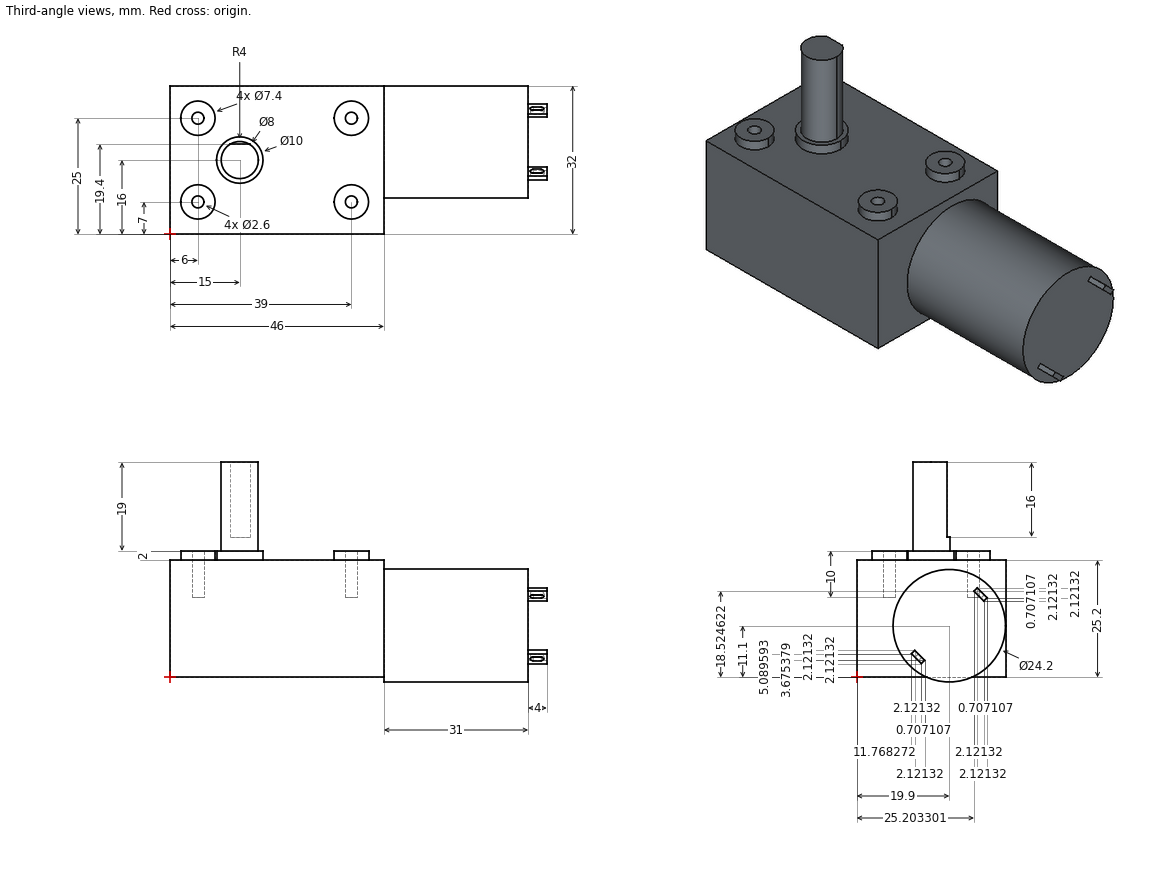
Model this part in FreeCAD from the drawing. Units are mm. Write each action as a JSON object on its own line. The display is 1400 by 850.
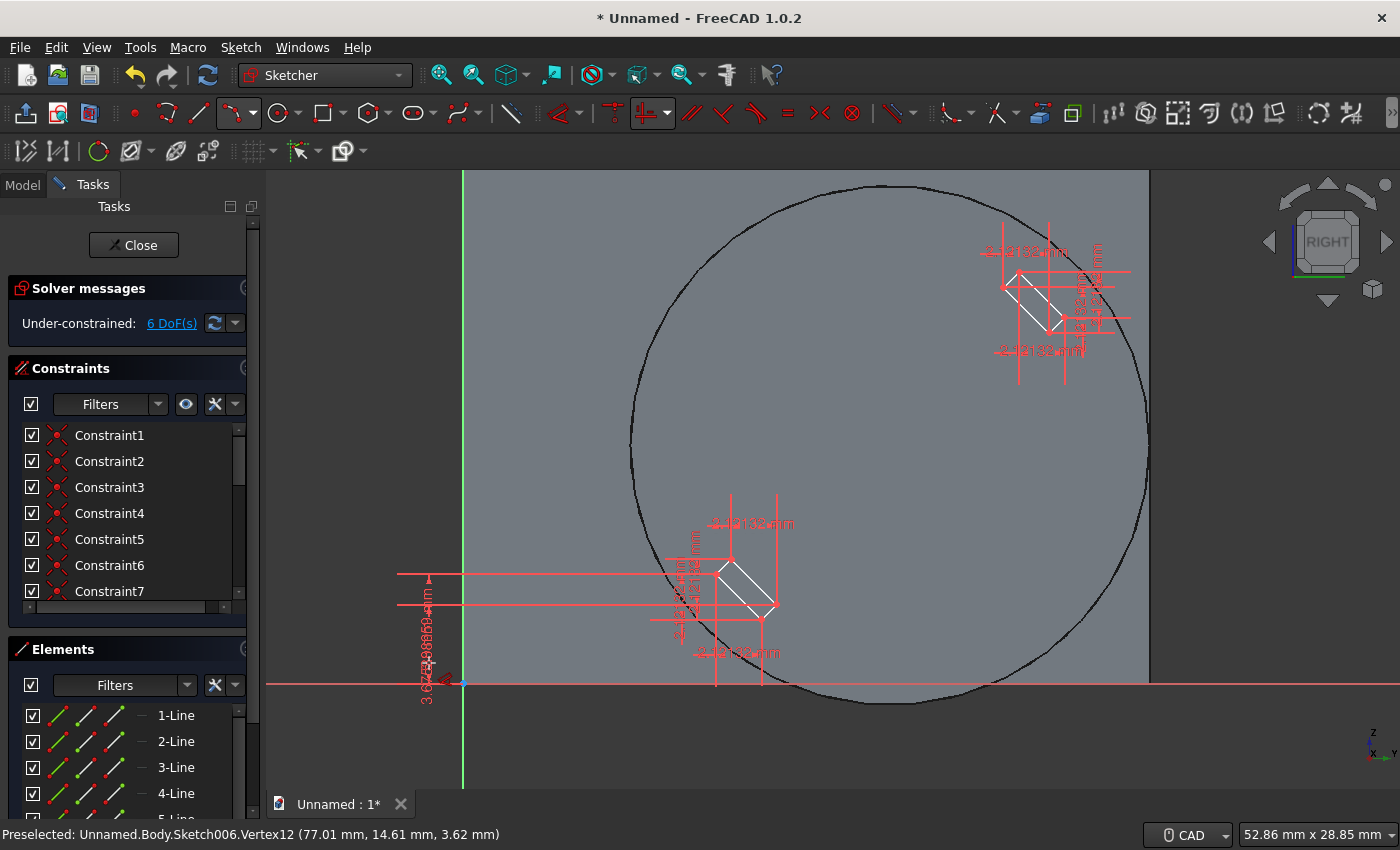
{"action": "scroll", "coordinate": [1057, 326], "scroll_direction": "up", "scroll_amount": 5}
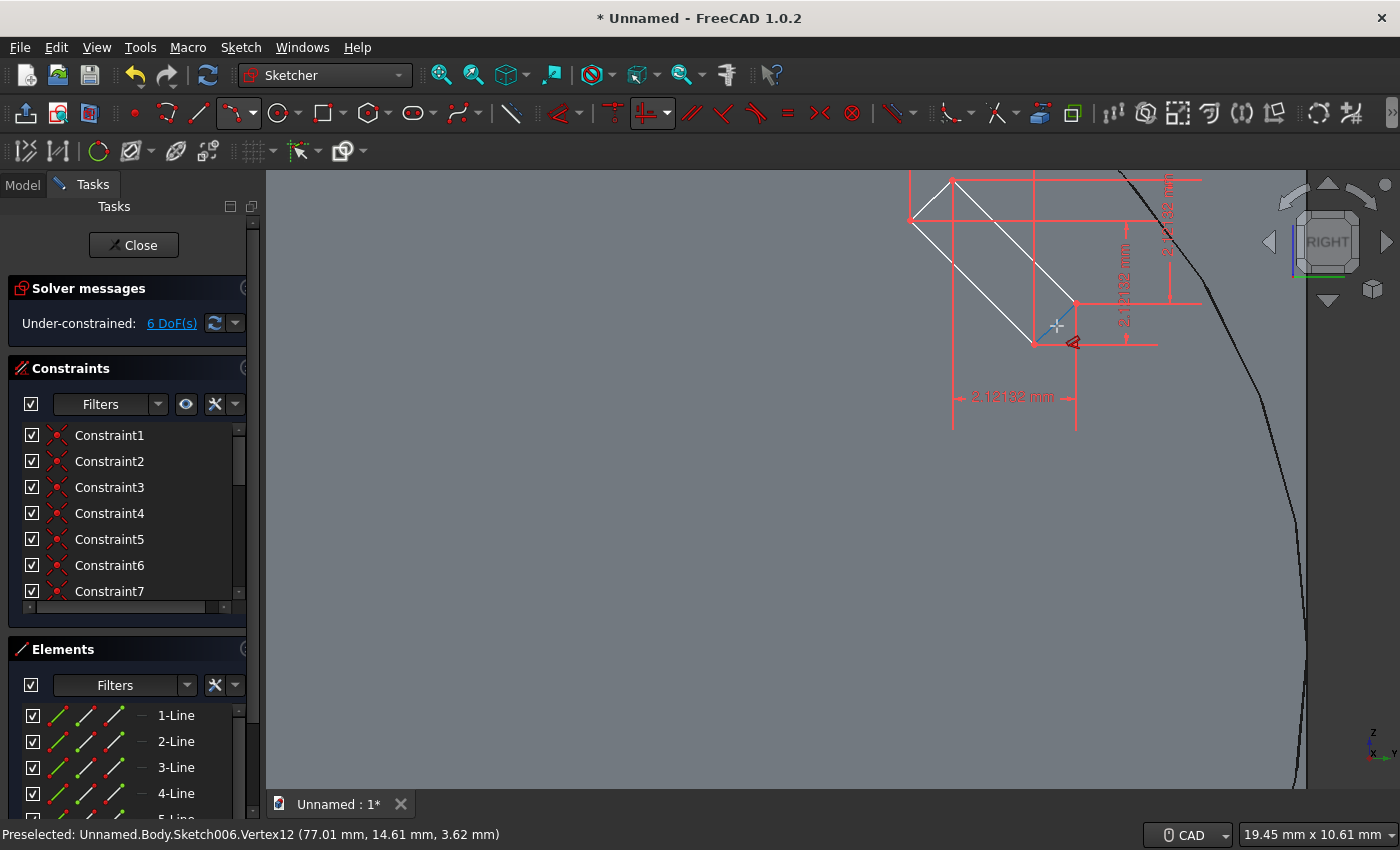
{"action": "left_click", "coordinate": [1055, 324]}
{"action": "left_click", "coordinate": [1055, 246]}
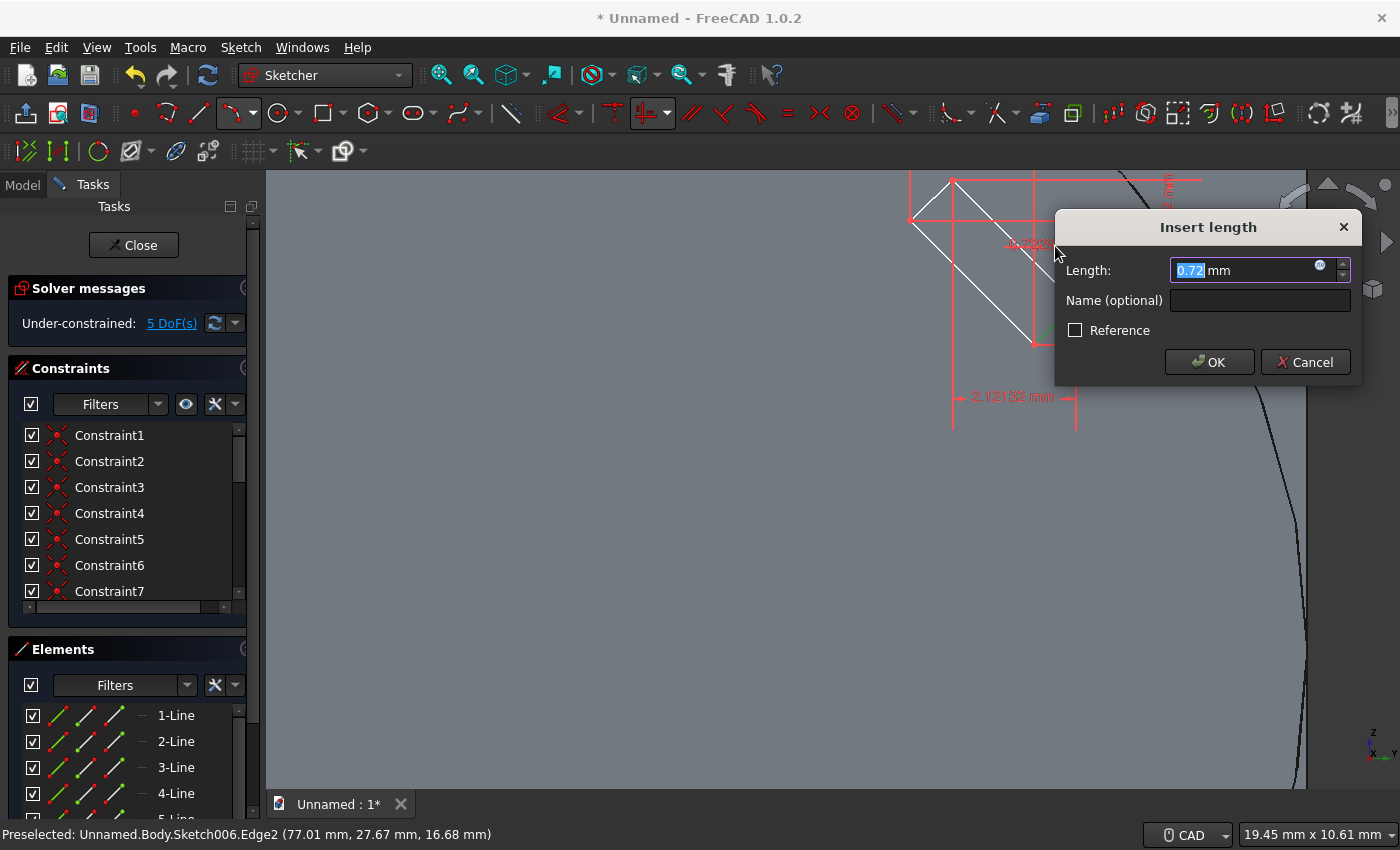
{"action": "type", "text": "0.707107"}
{"action": "key", "text": "Return"}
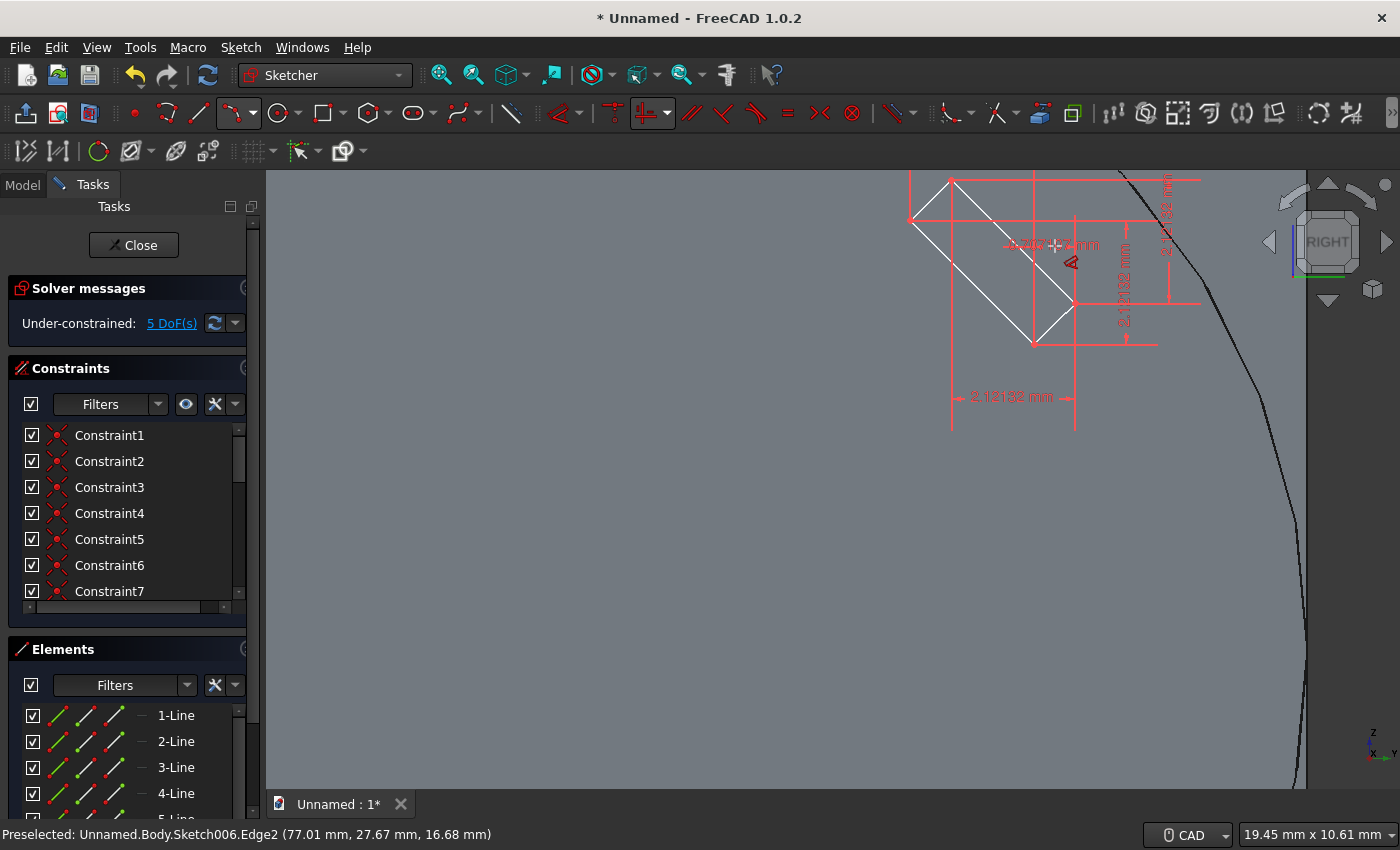
{"action": "left_click", "coordinate": [1046, 332]}
{"action": "left_click", "coordinate": [1109, 324]}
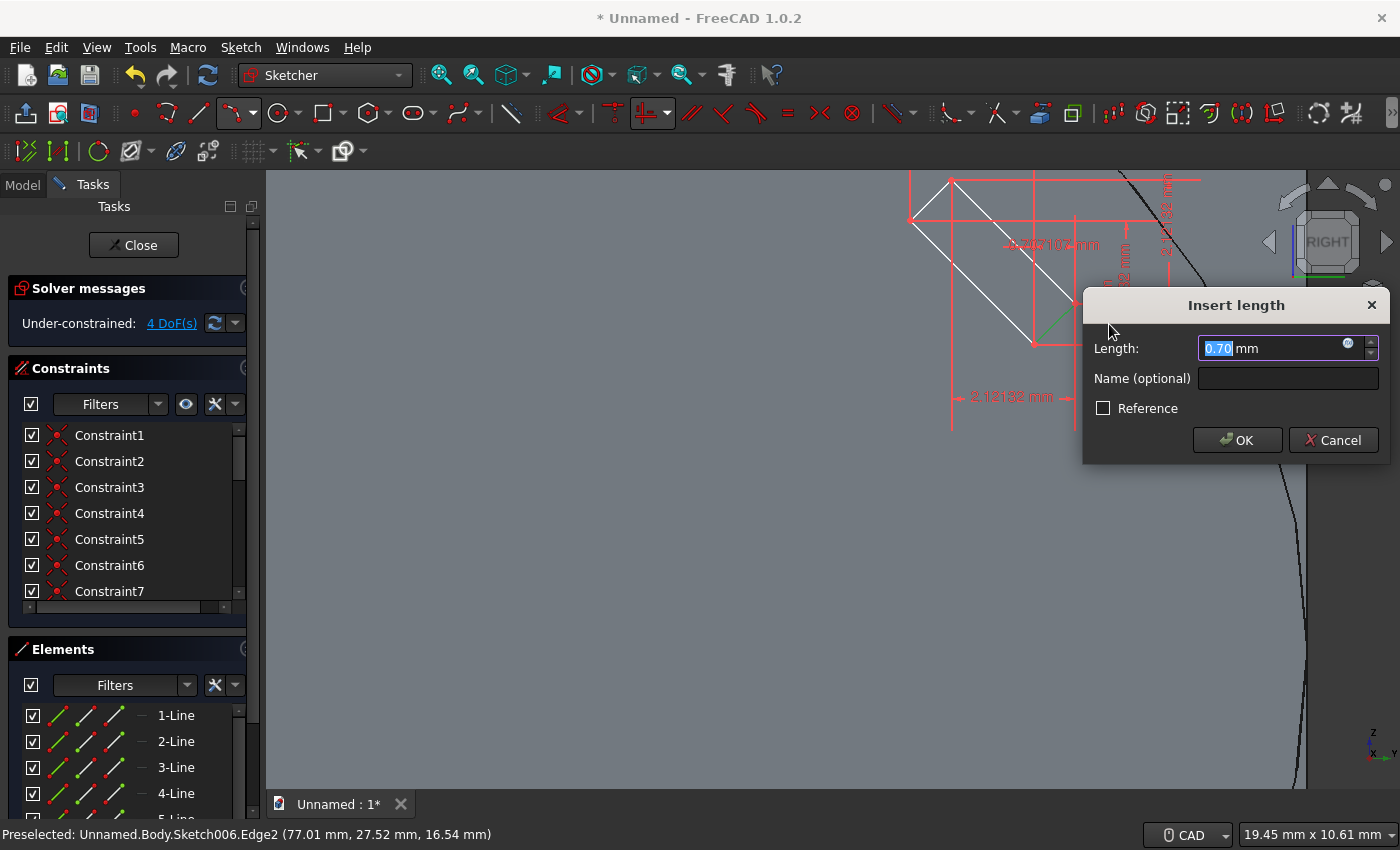
{"action": "type", "text": "0.707107"}
{"action": "key", "text": "Return"}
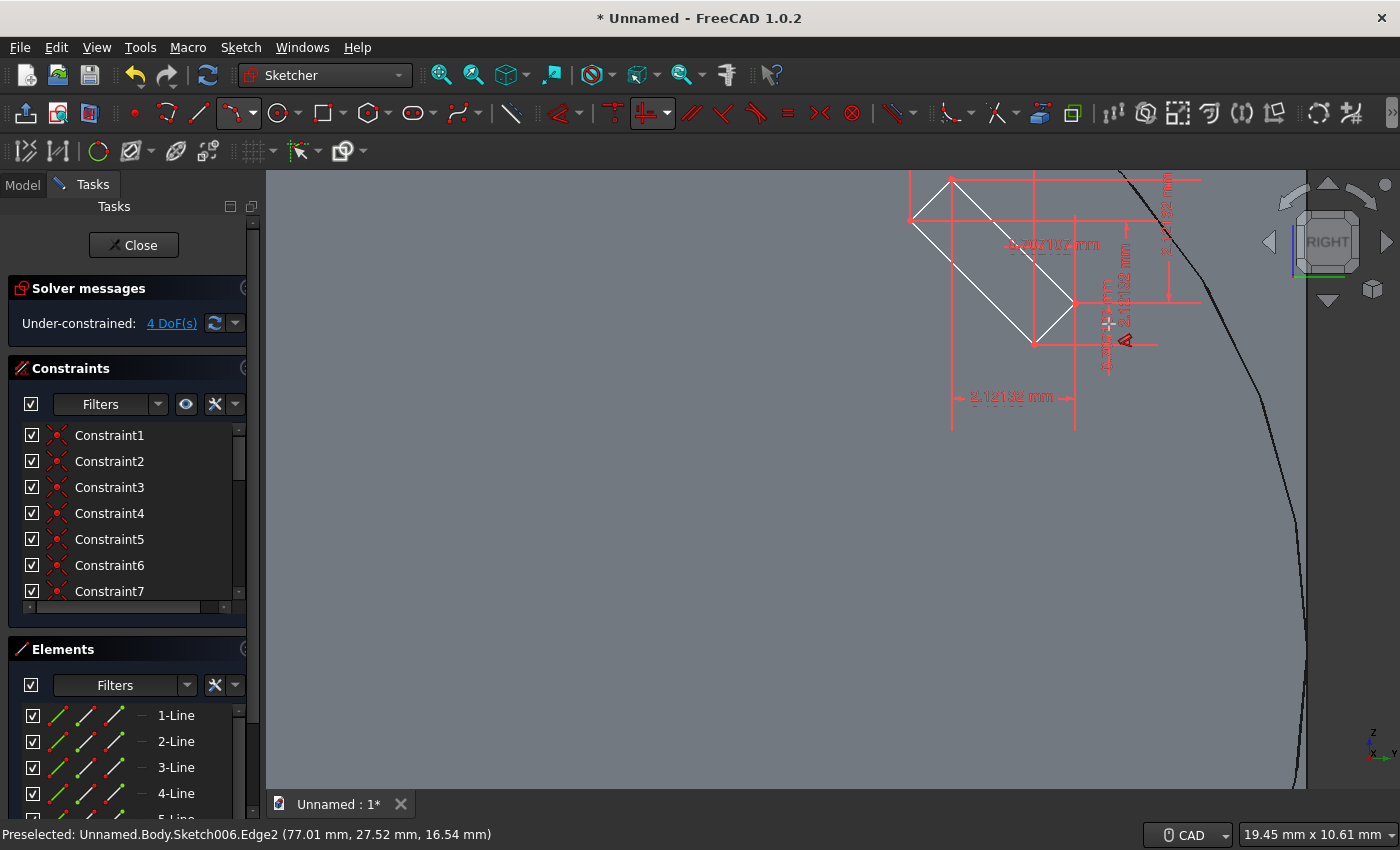
{"action": "scroll", "coordinate": [1059, 330], "scroll_direction": "down", "scroll_amount": 5}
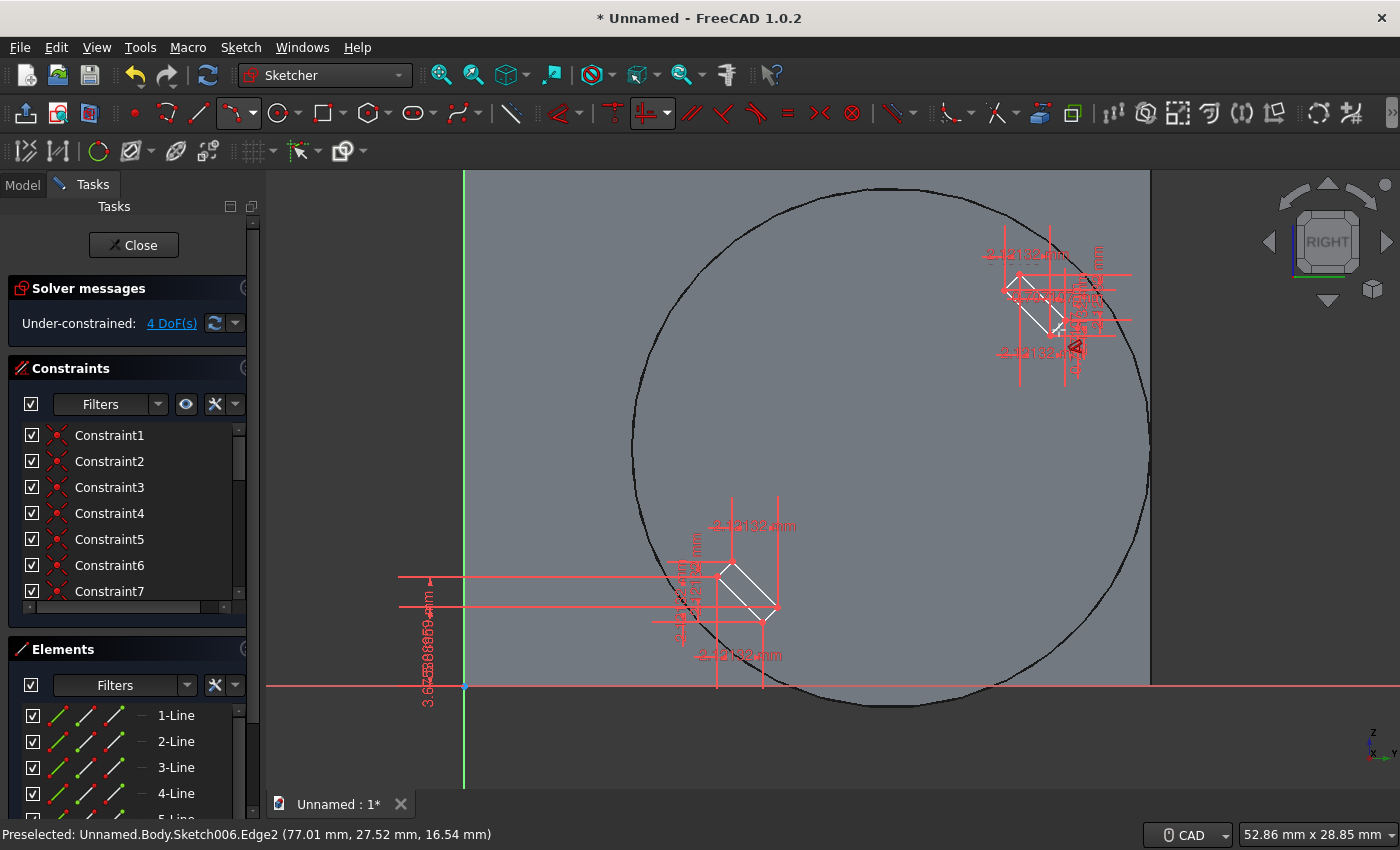
{"action": "scroll", "coordinate": [767, 618], "scroll_direction": "up", "scroll_amount": 5}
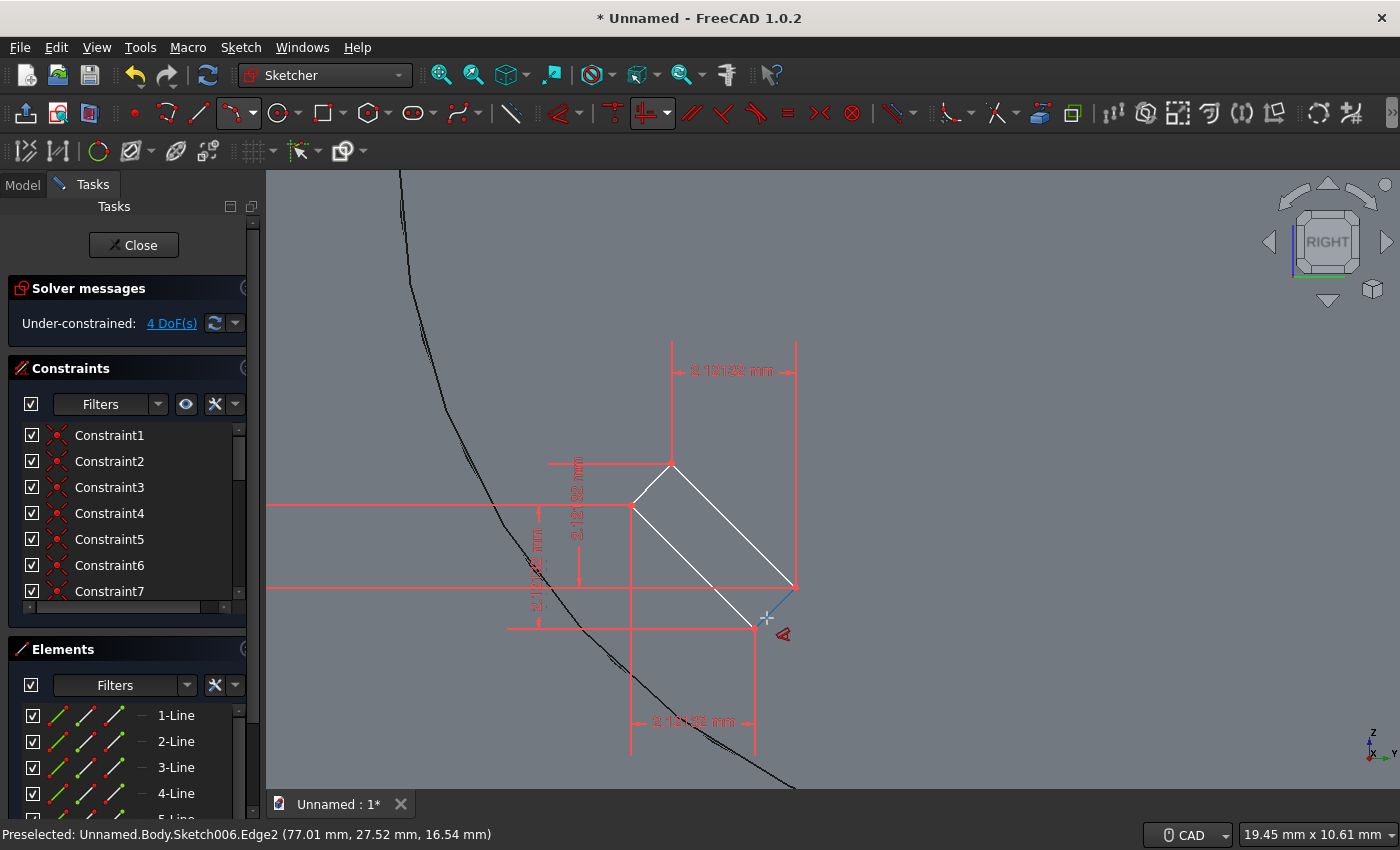
{"action": "left_click", "coordinate": [767, 616]}
{"action": "left_click", "coordinate": [775, 663]}